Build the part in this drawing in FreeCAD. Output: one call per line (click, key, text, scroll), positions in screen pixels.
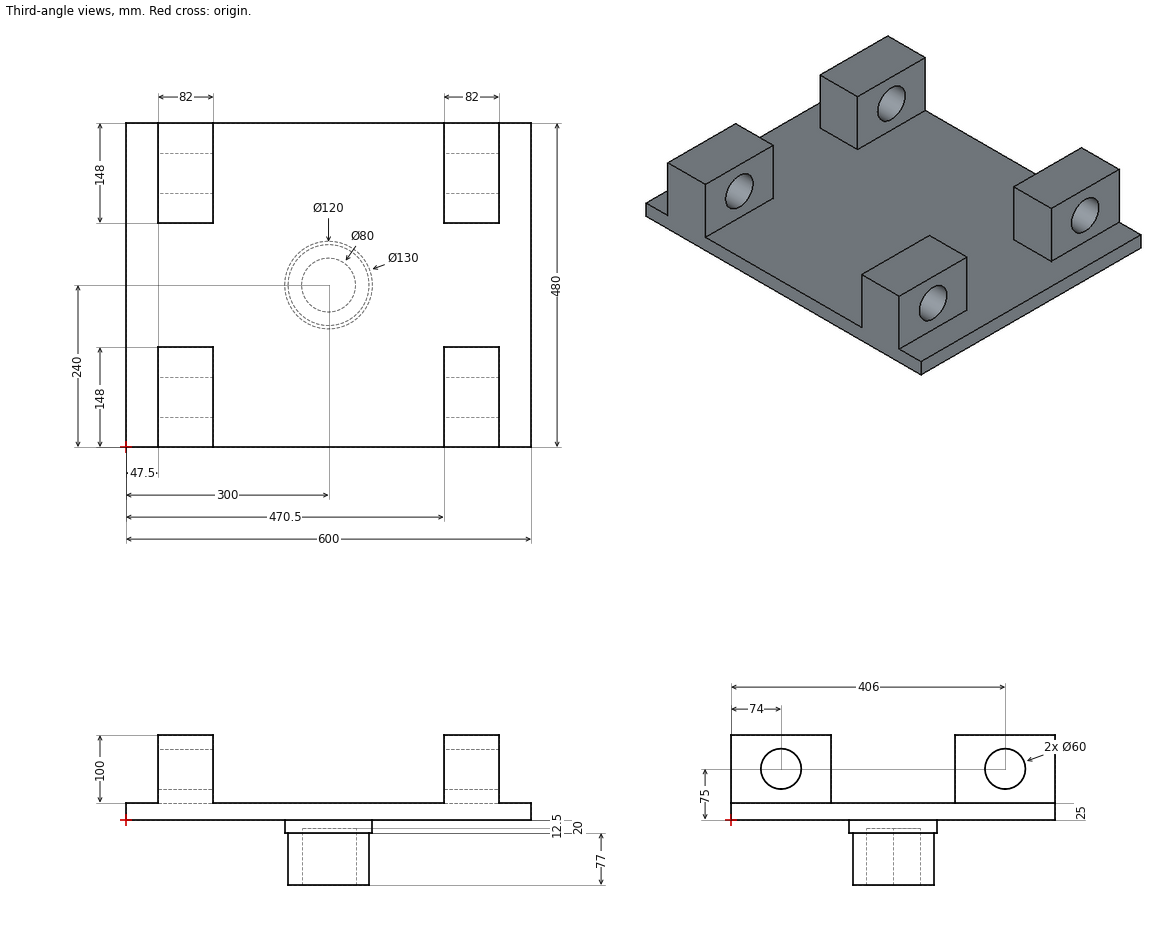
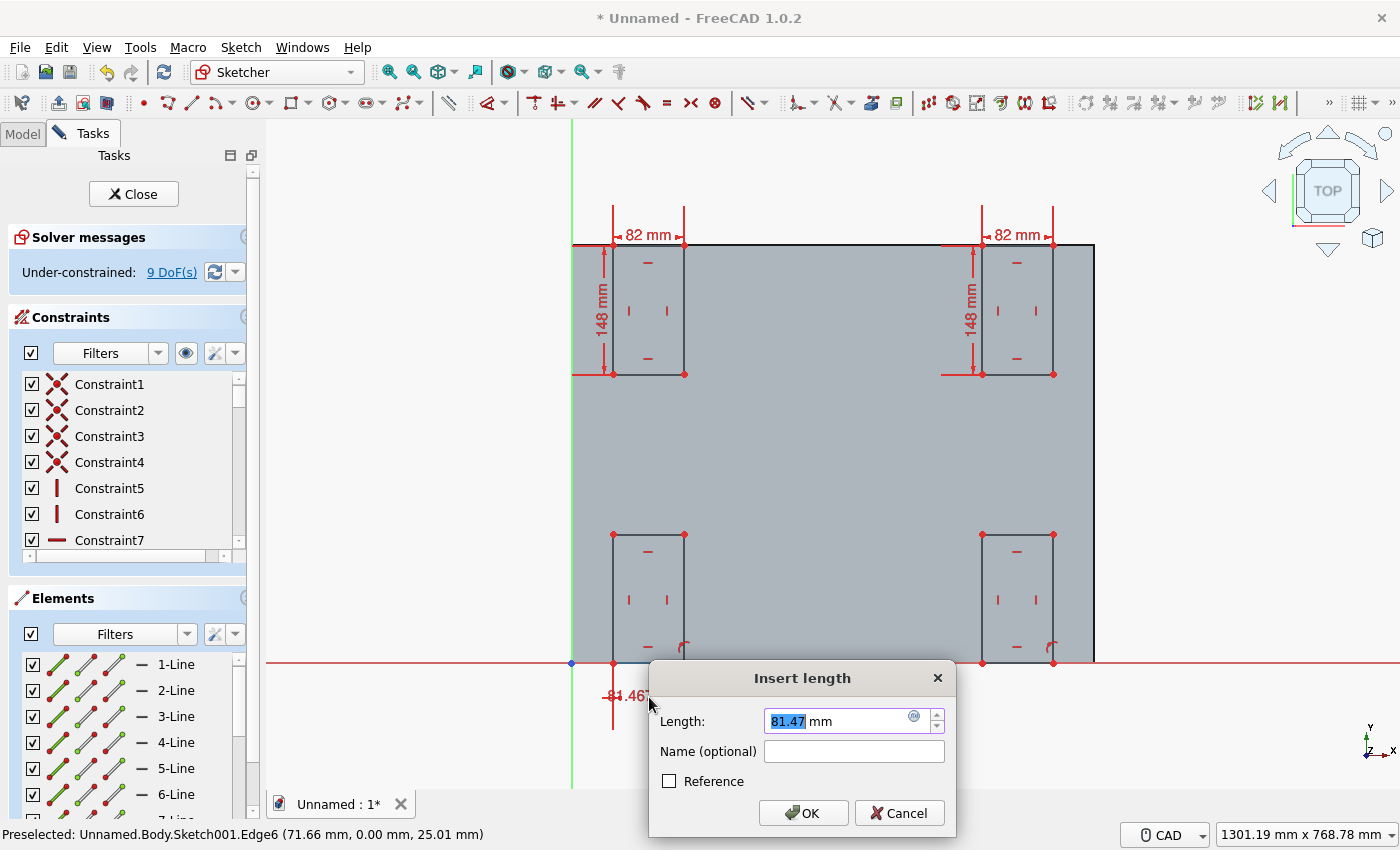
text(82)
key(Return)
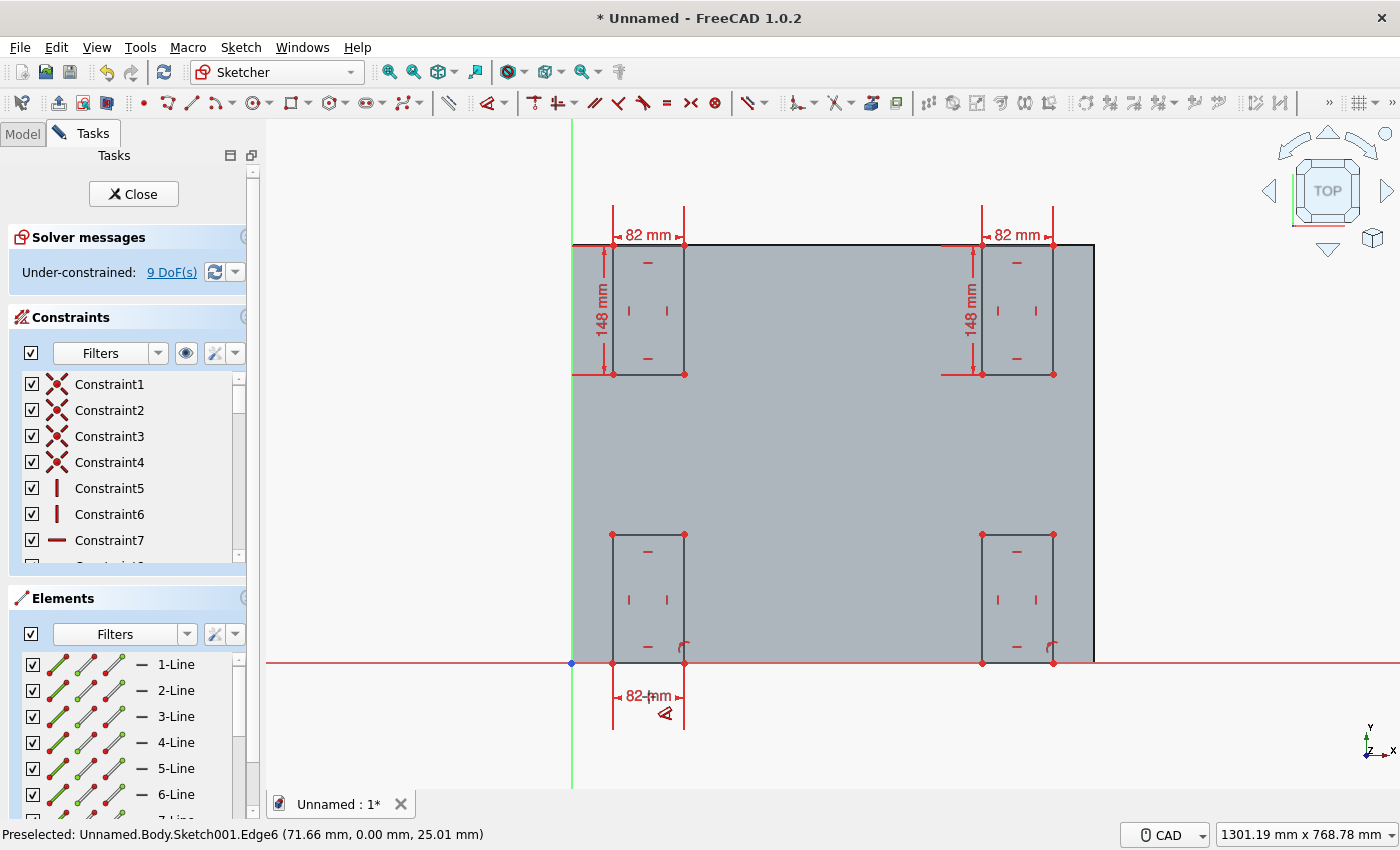
click(1003, 663)
click(1017, 697)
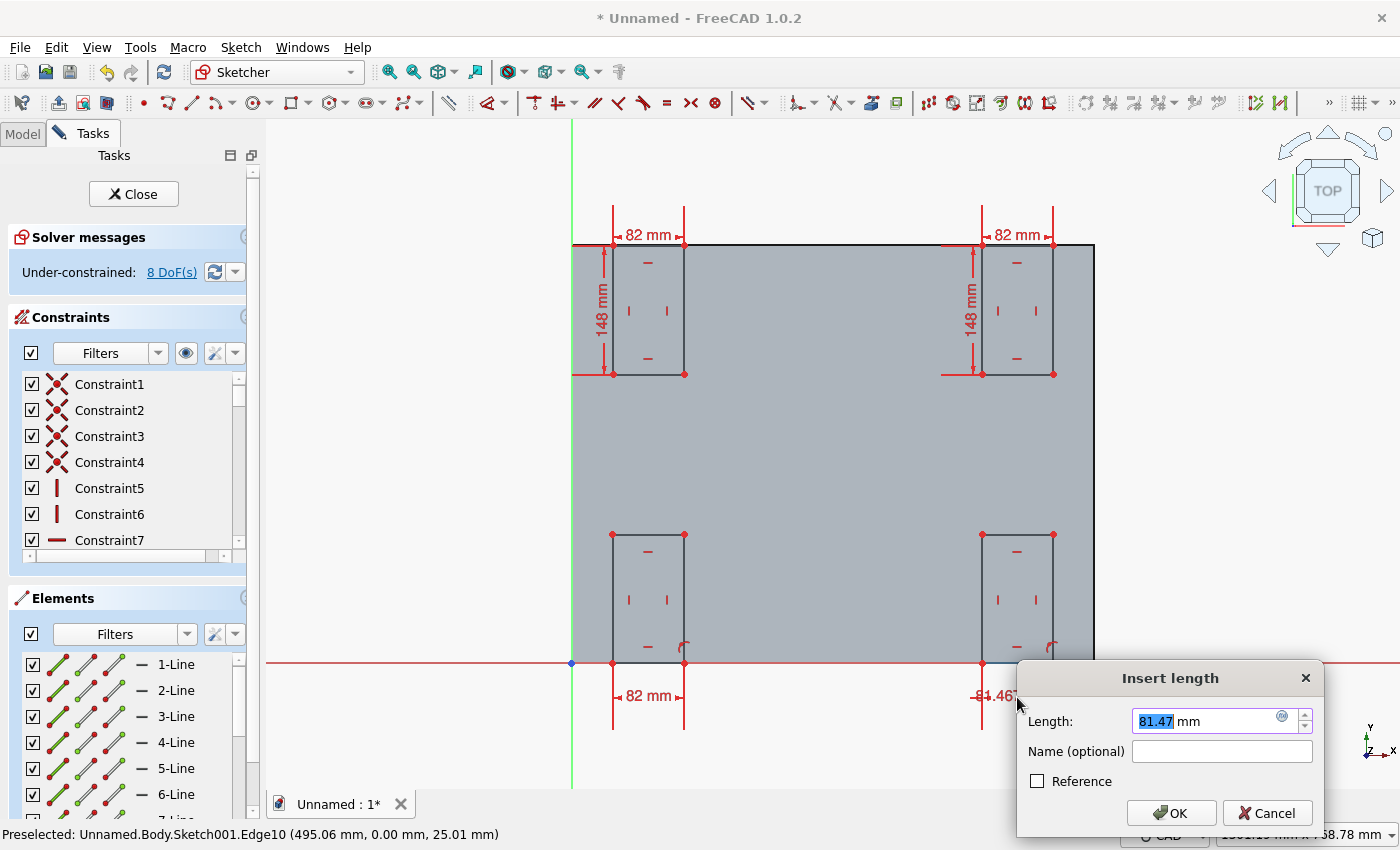
text(82)
key(Return)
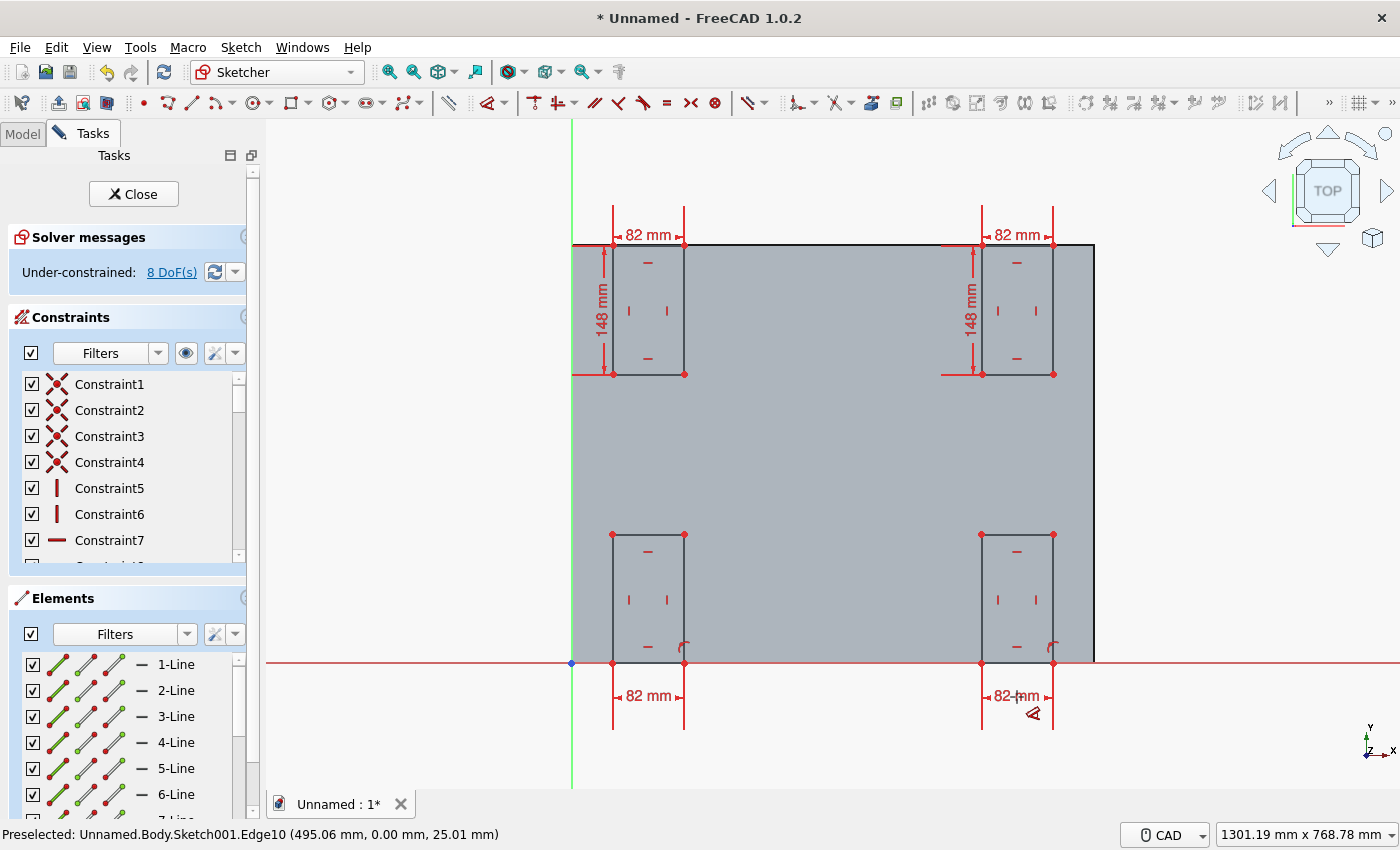
click(613, 573)
click(647, 599)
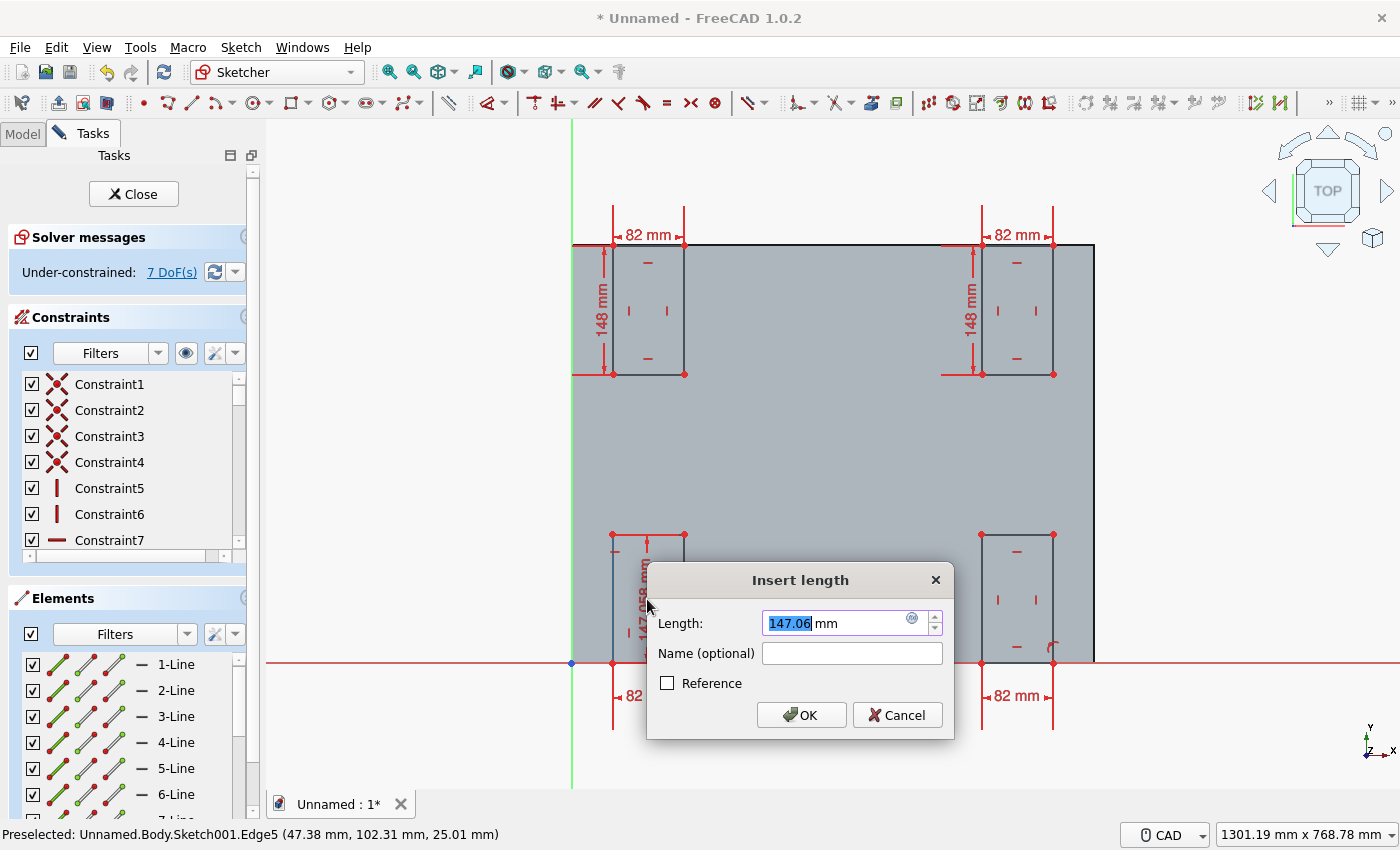
text(148)
key(Return)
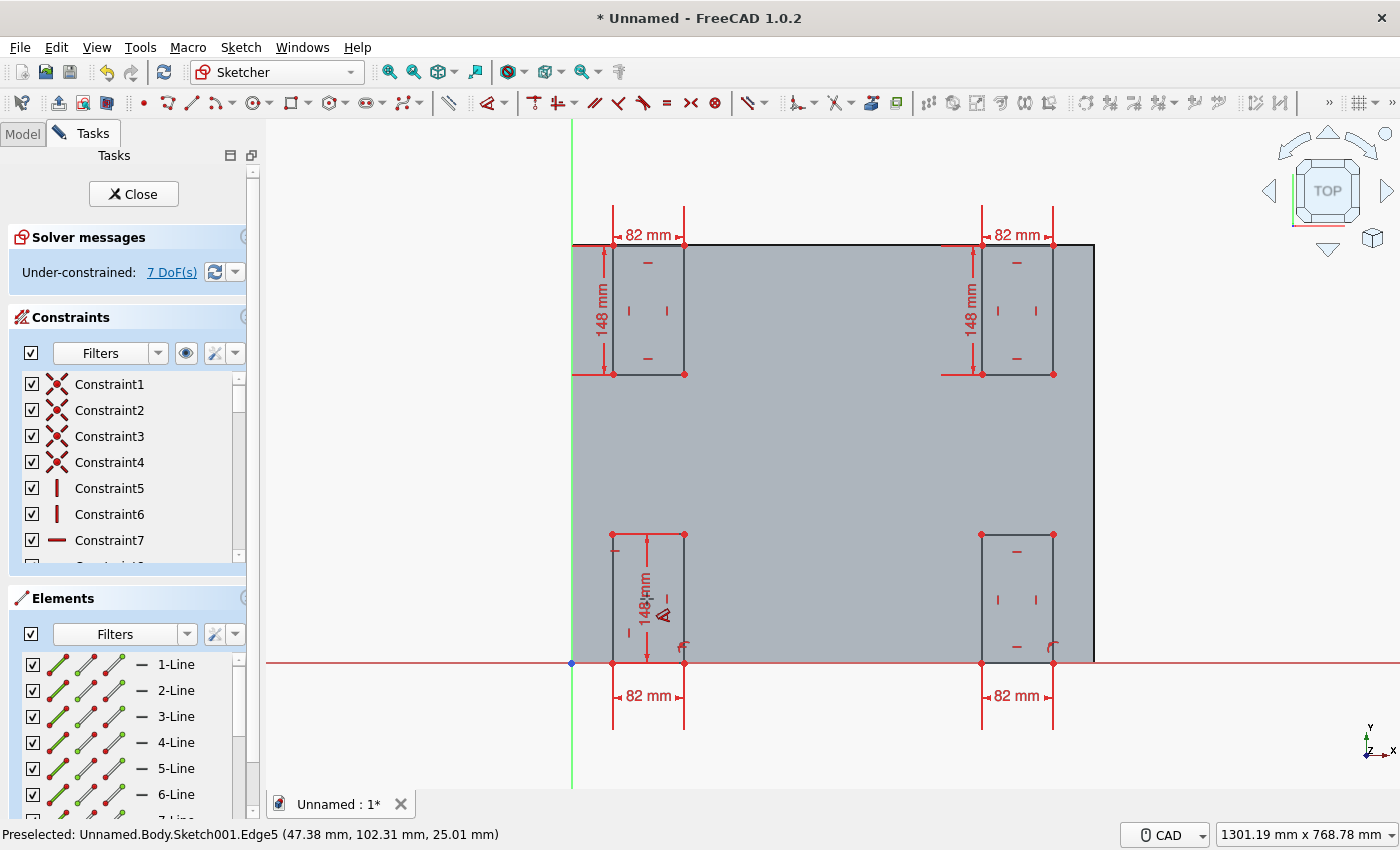
click(982, 573)
click(1016, 599)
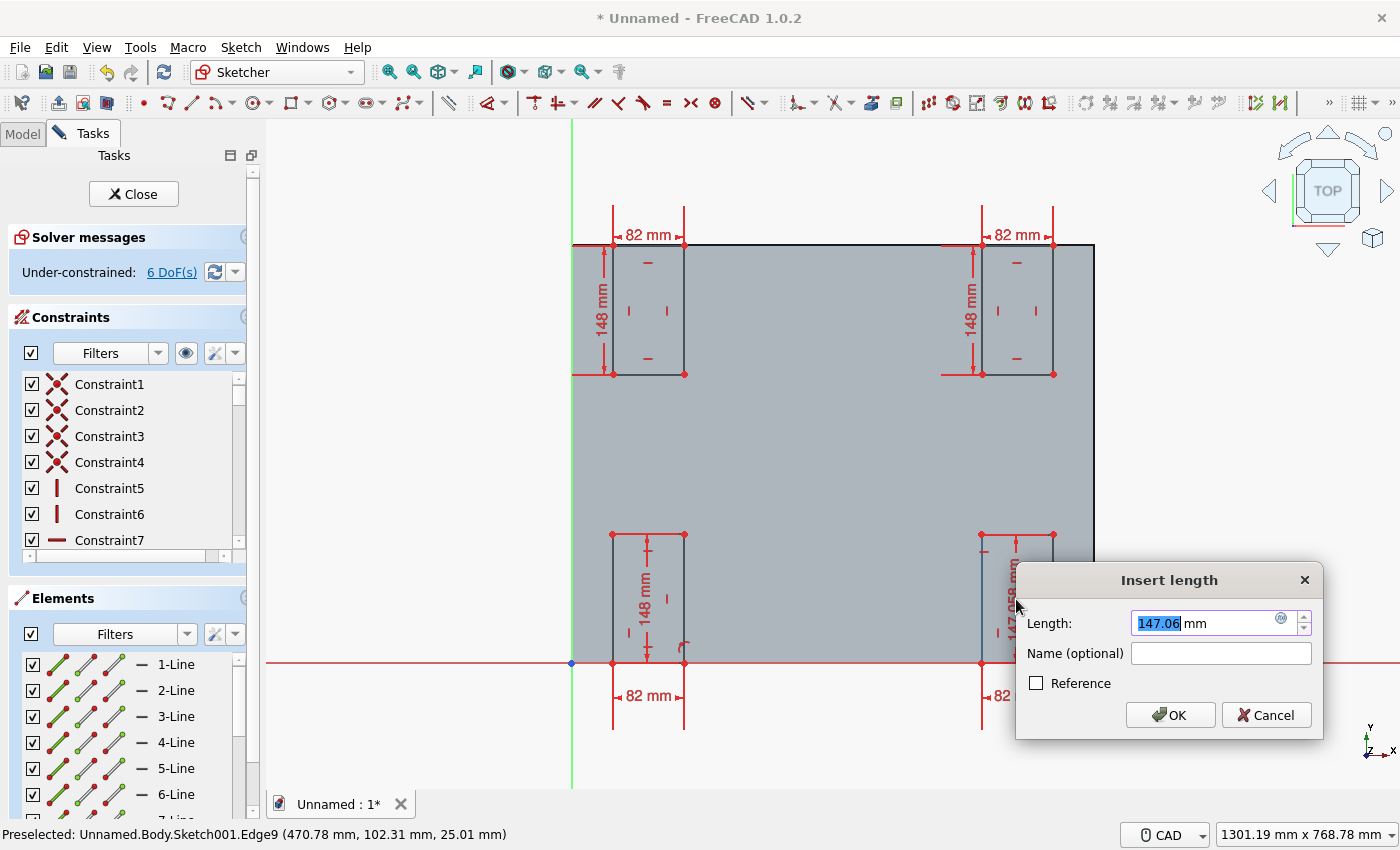
text(148)
key(Return)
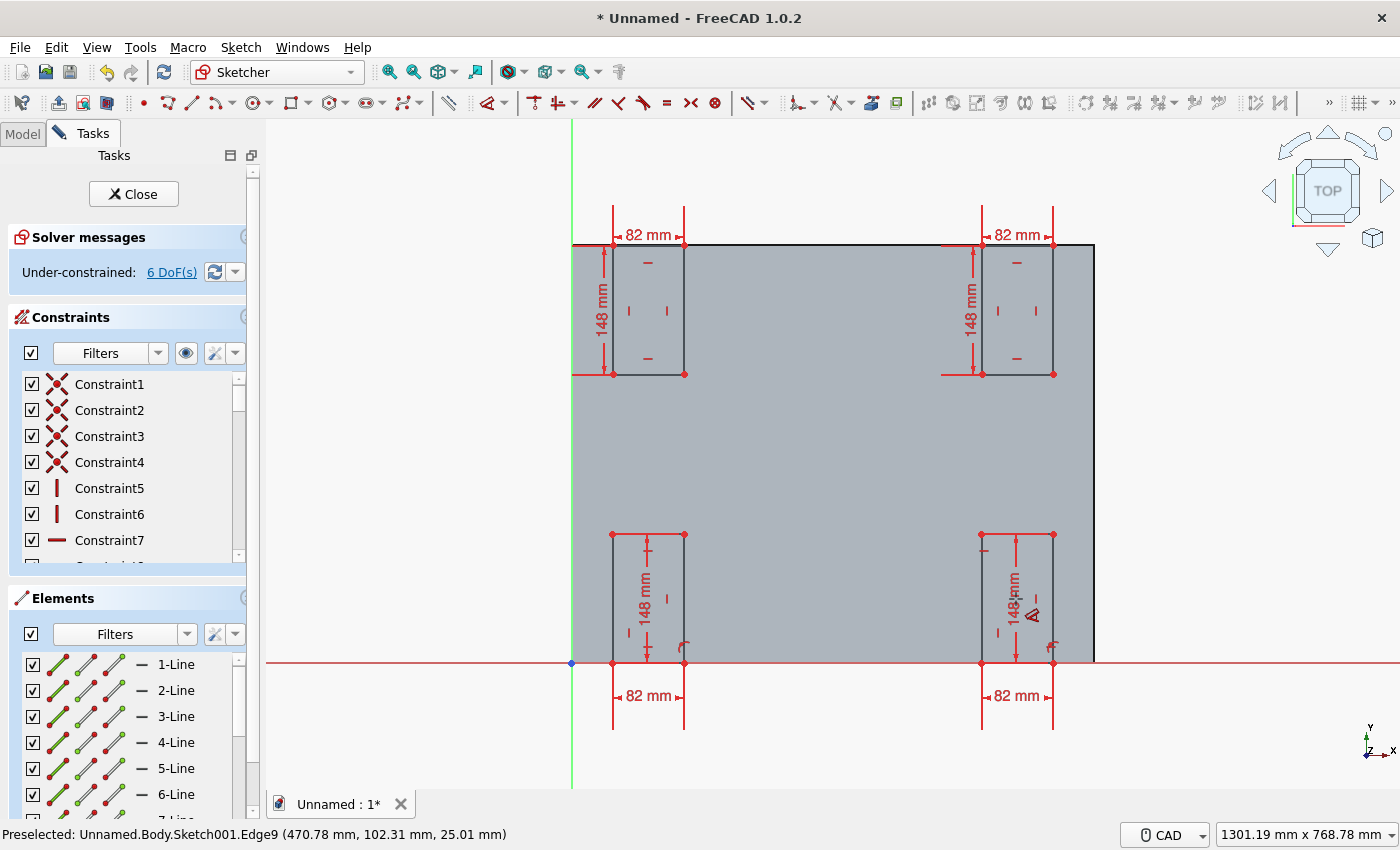
click(613, 246)
click(538, 455)